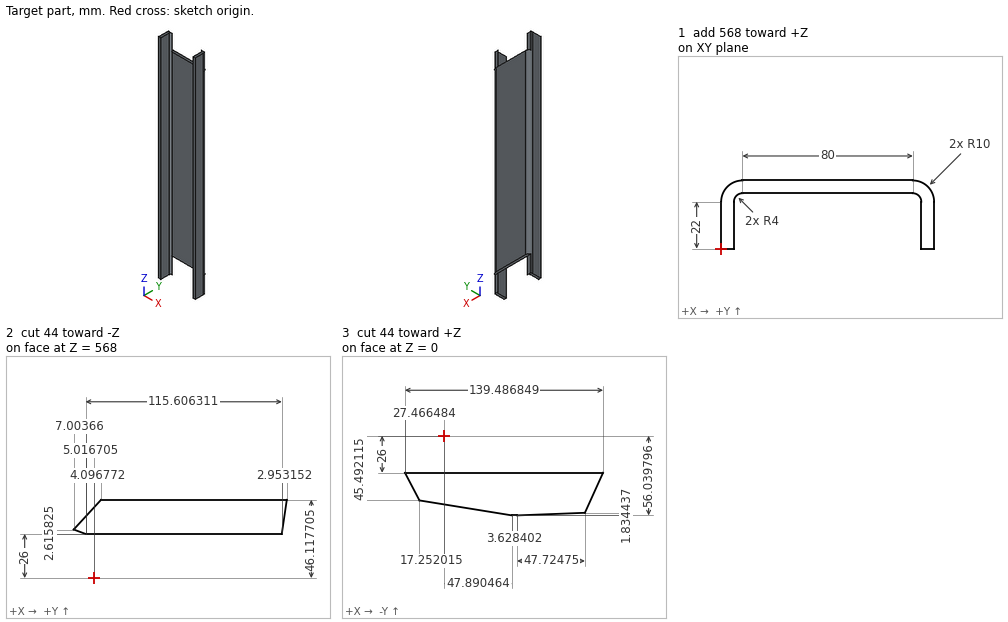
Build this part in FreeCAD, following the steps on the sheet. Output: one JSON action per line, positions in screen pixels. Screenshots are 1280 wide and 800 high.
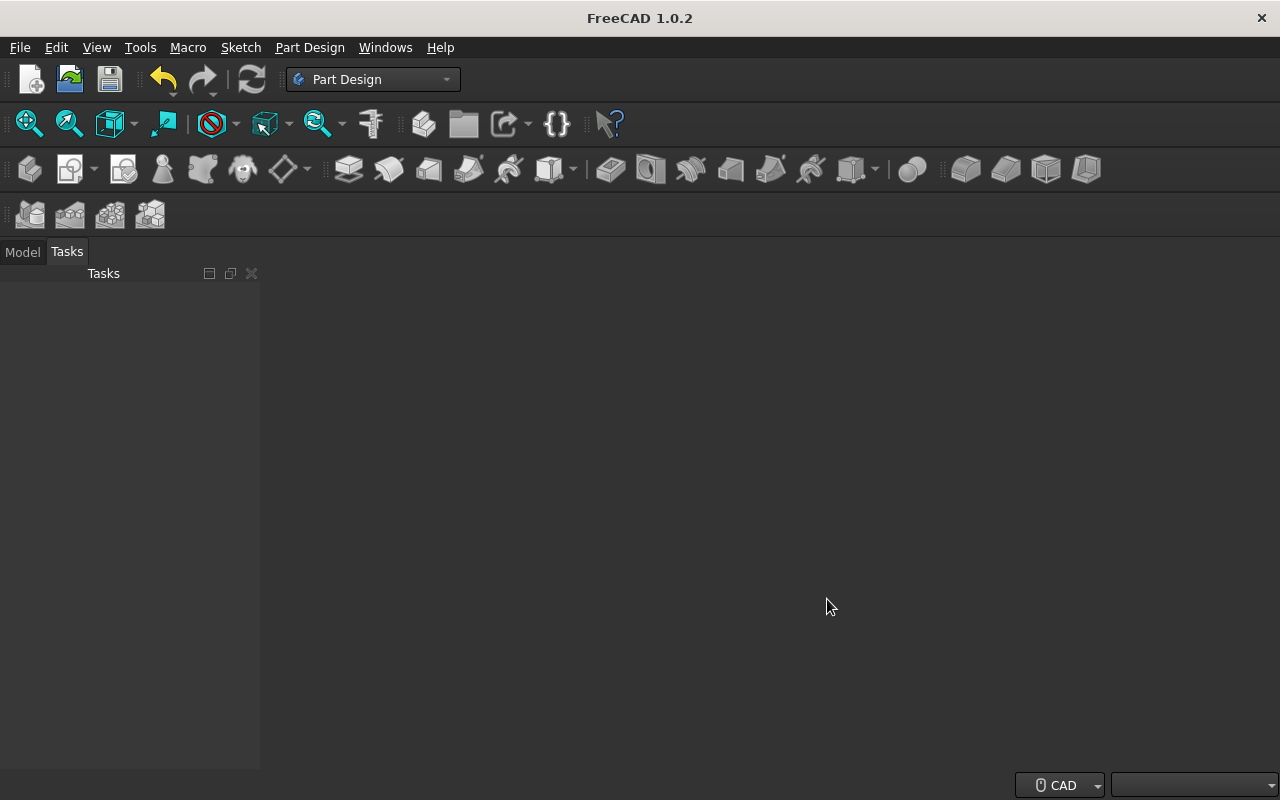
{"action": "left_click", "coordinate": [30, 80]}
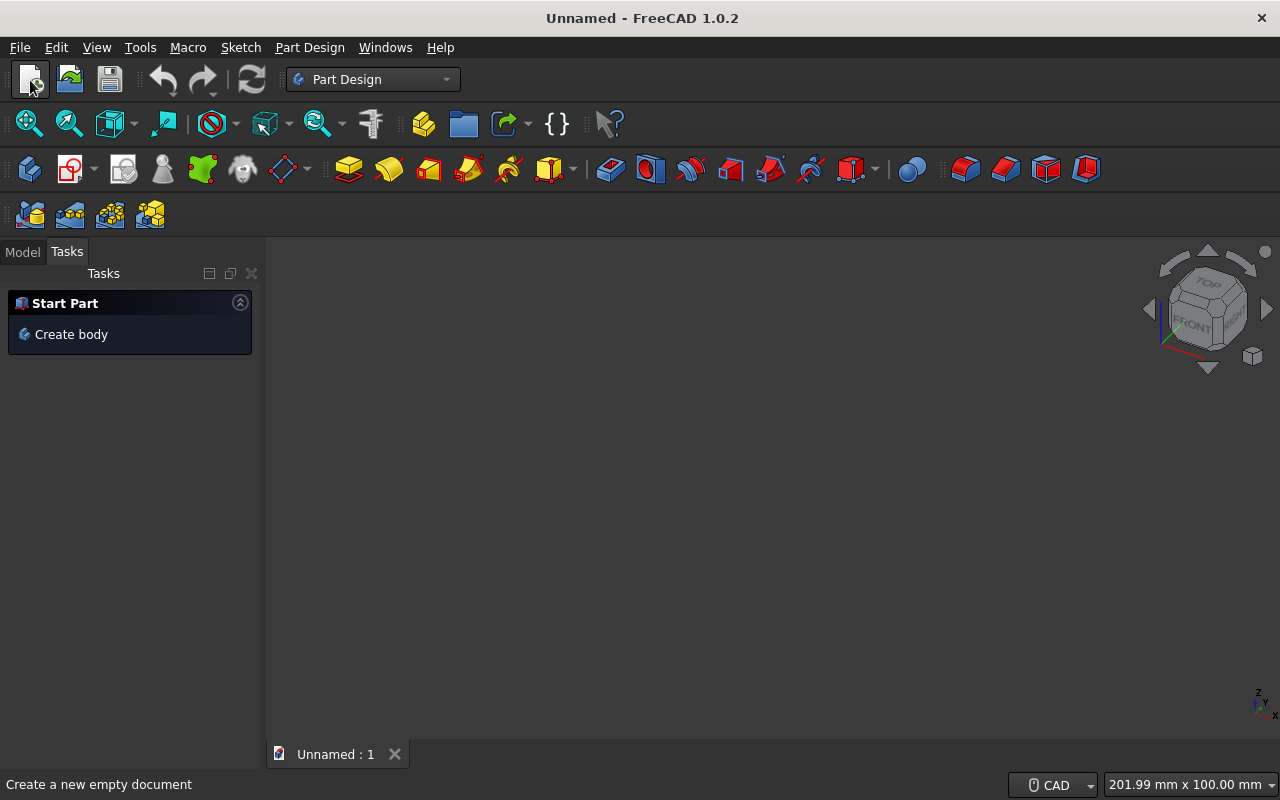
{"action": "left_click", "coordinate": [70, 170]}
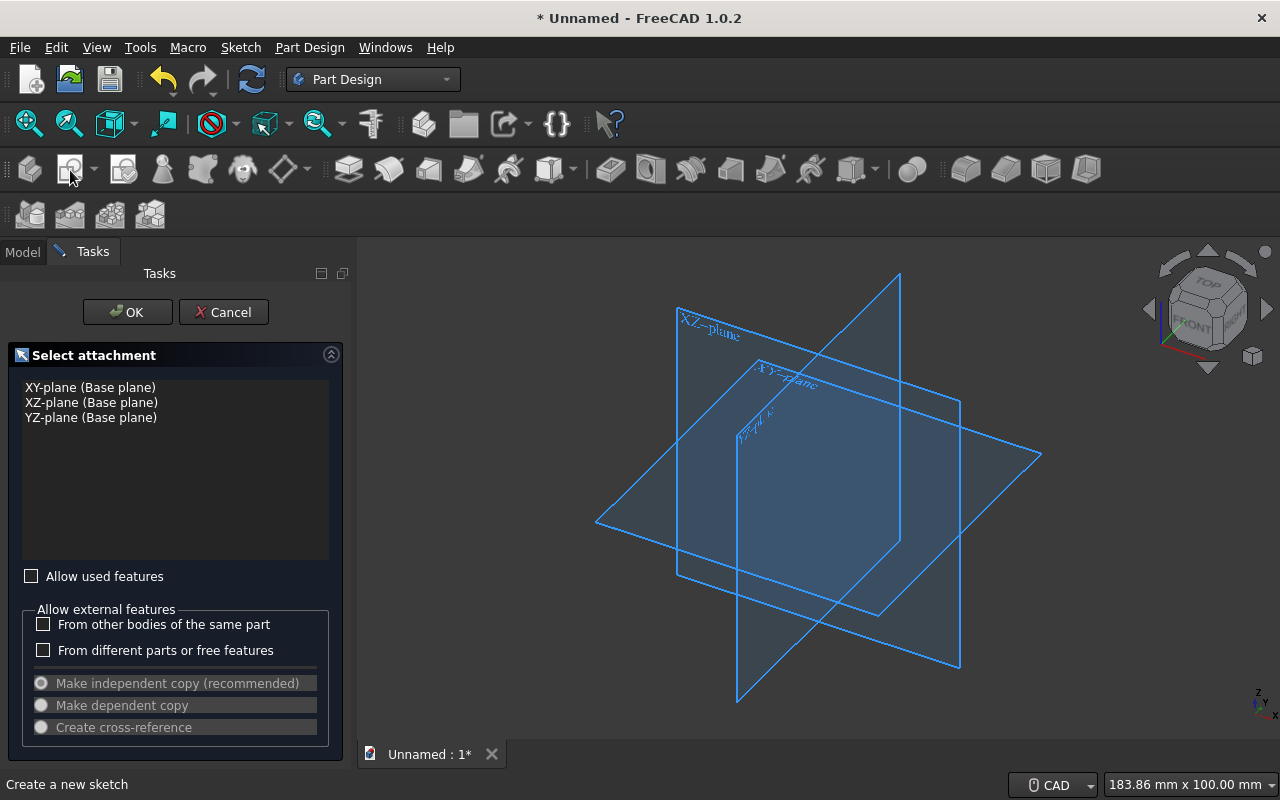
{"action": "left_click", "coordinate": [82, 388]}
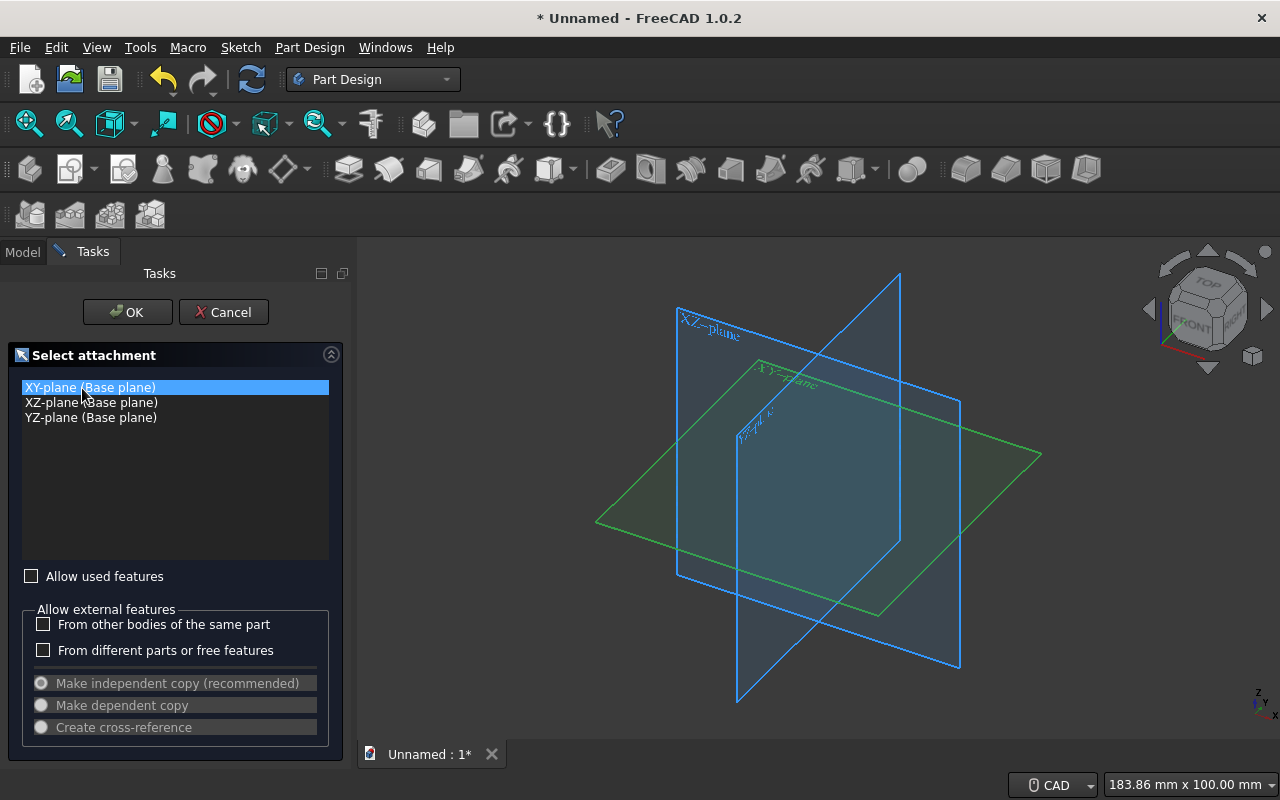
{"action": "left_click", "coordinate": [128, 312]}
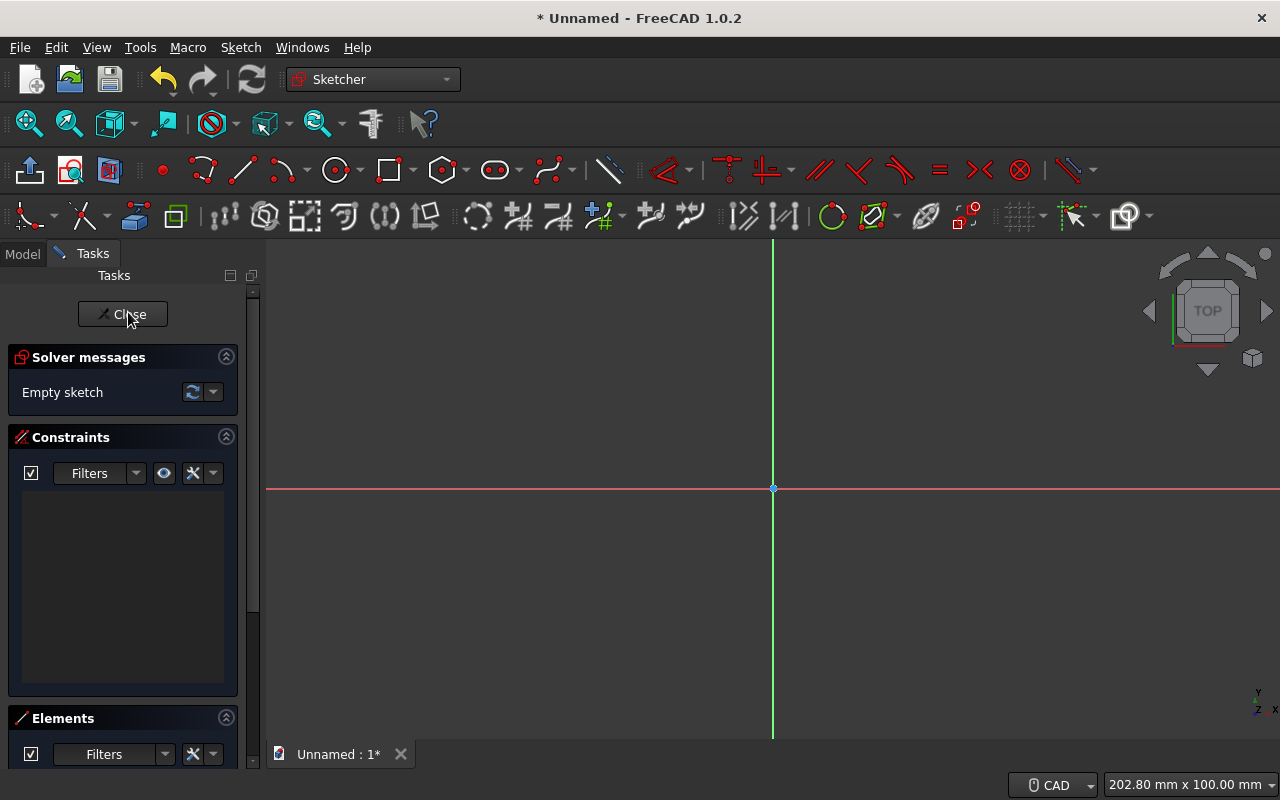
{"action": "scroll", "coordinate": [294, 652], "scroll_direction": "down", "scroll_amount": 2}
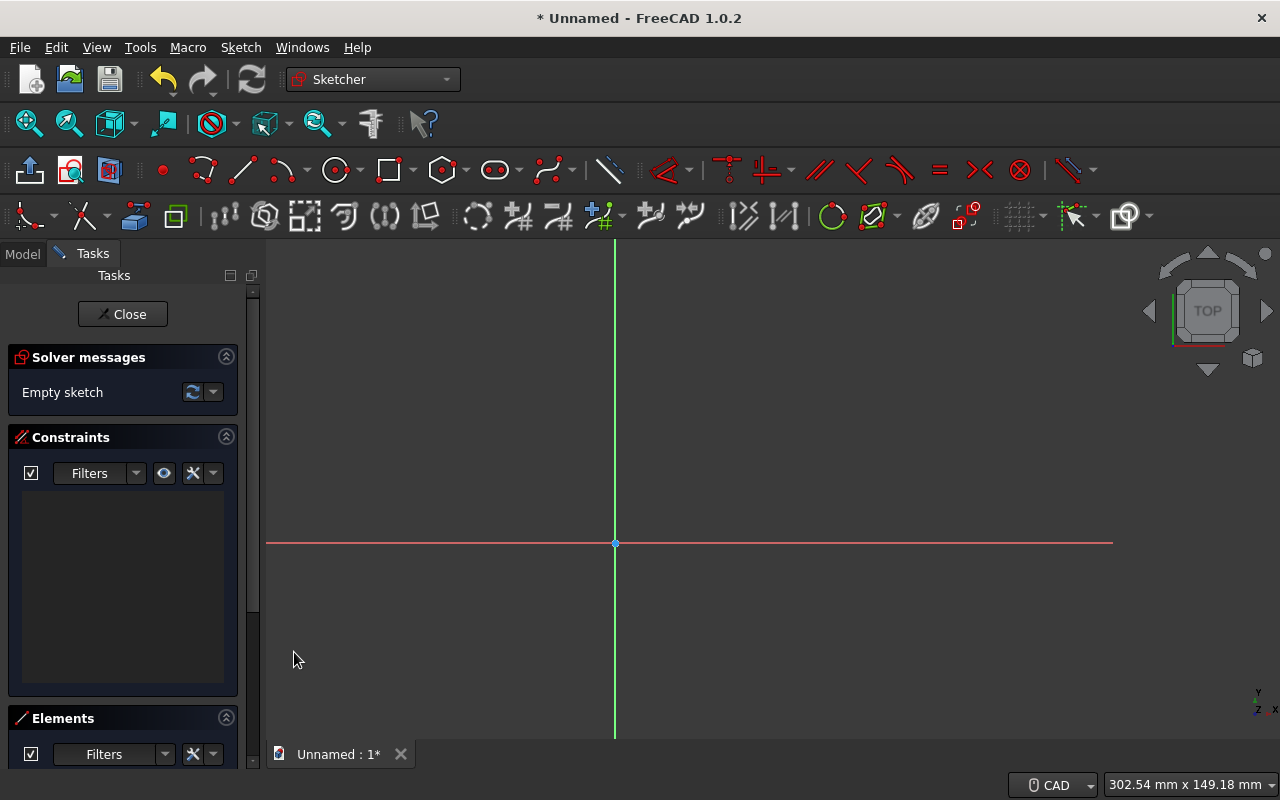
{"action": "scroll", "coordinate": [878, 490], "scroll_direction": "up", "scroll_amount": 3}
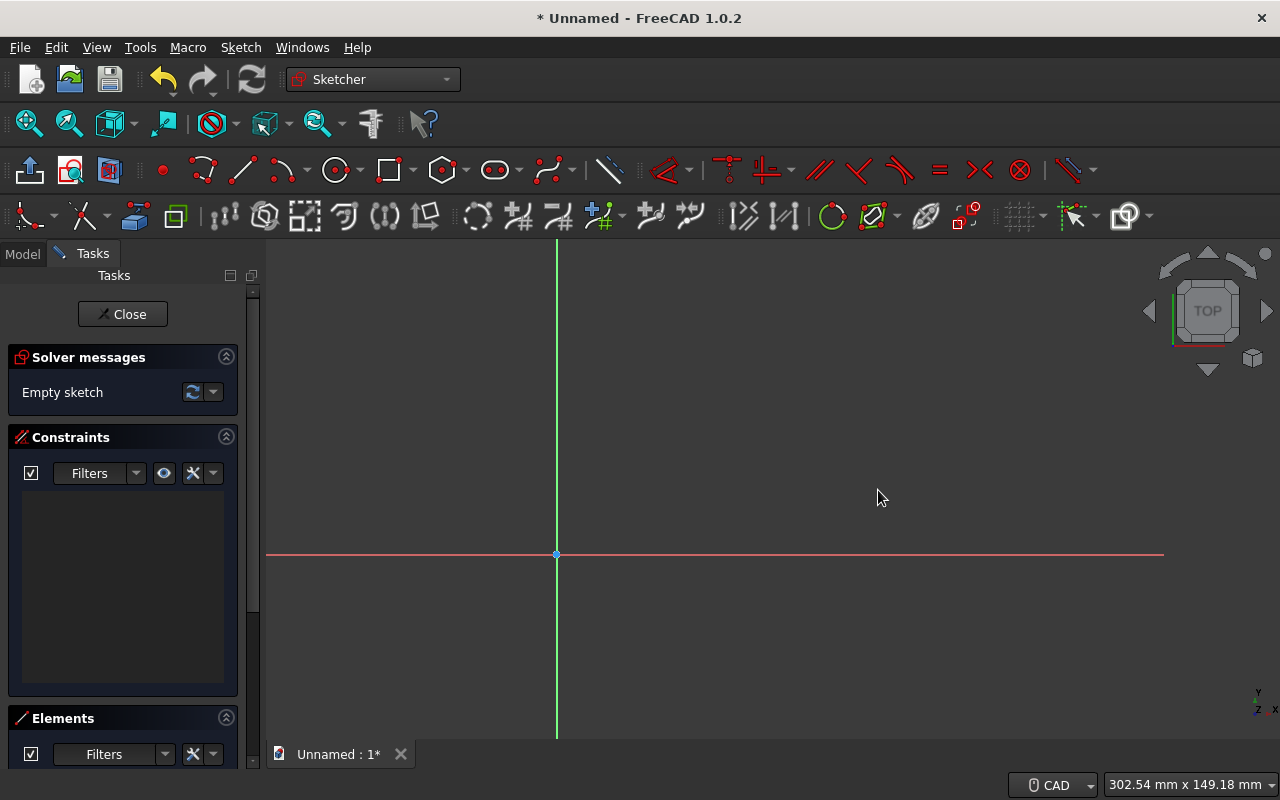
{"action": "left_click", "coordinate": [204, 170]}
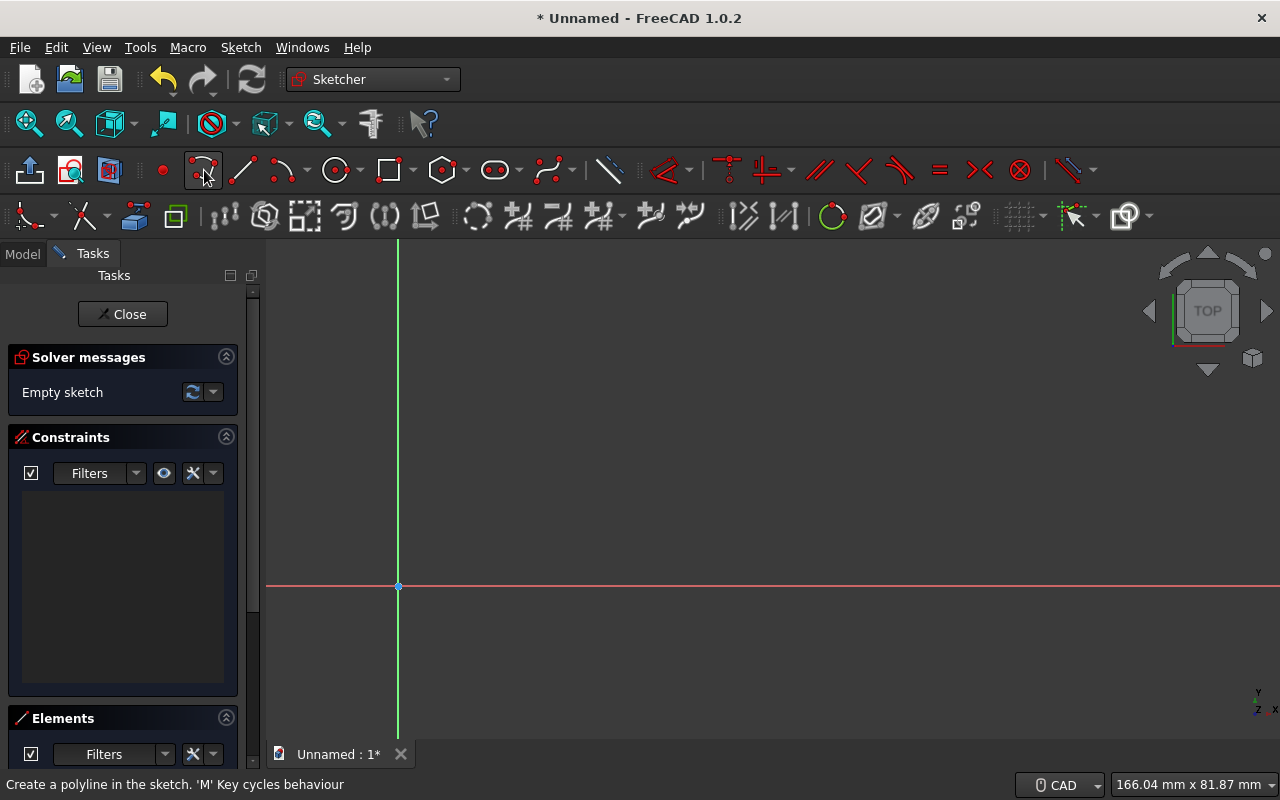
{"action": "left_click", "coordinate": [398, 452]}
{"action": "left_click", "coordinate": [398, 586]}
{"action": "left_click", "coordinate": [435, 577]}
{"action": "left_click", "coordinate": [435, 452]}
{"action": "right_click", "coordinate": [435, 452]}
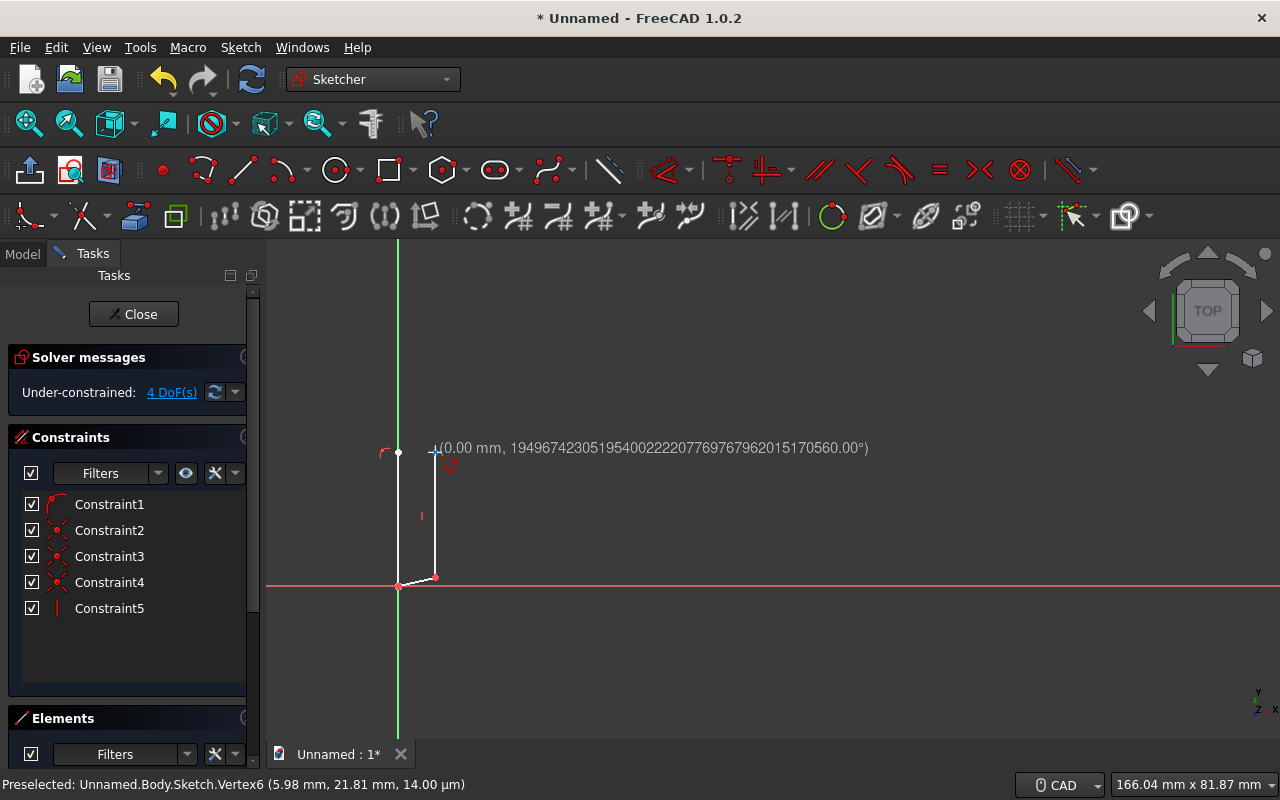
{"action": "left_click", "coordinate": [244, 170]}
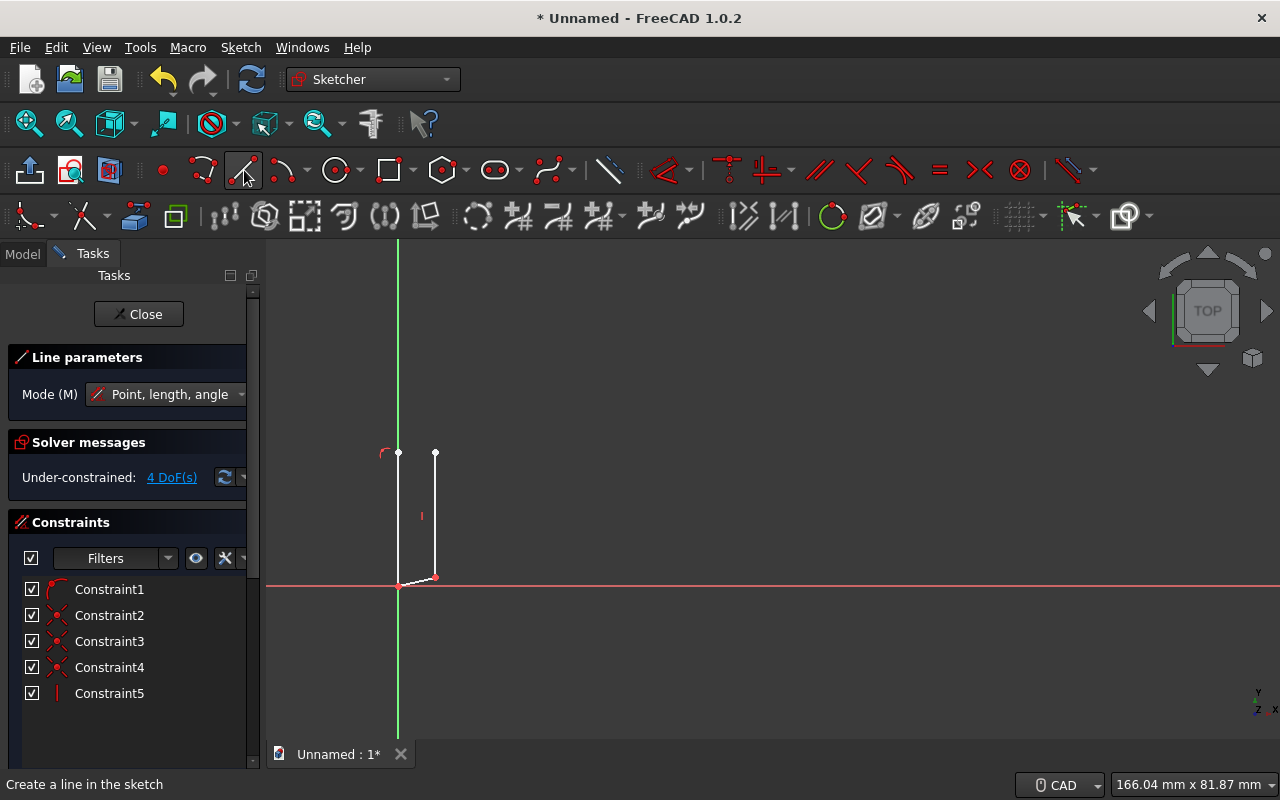
{"action": "left_click", "coordinate": [460, 427]}
{"action": "left_click", "coordinate": [948, 427]}